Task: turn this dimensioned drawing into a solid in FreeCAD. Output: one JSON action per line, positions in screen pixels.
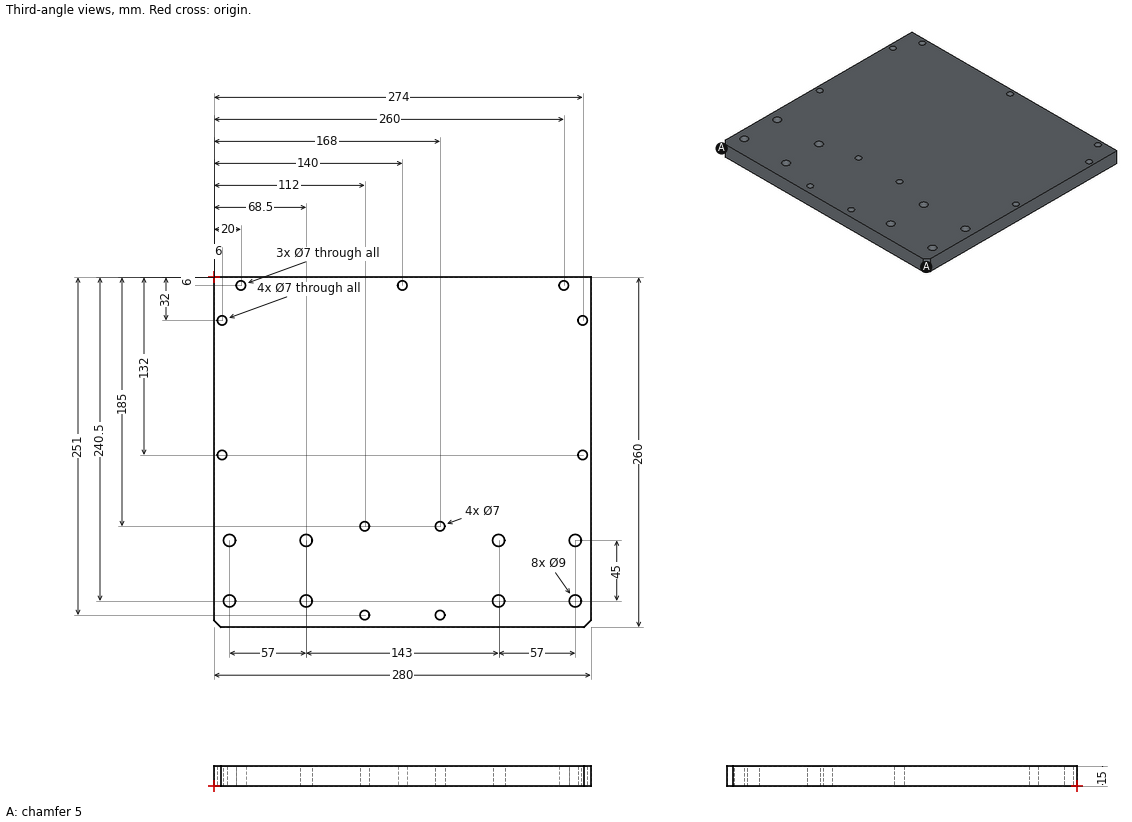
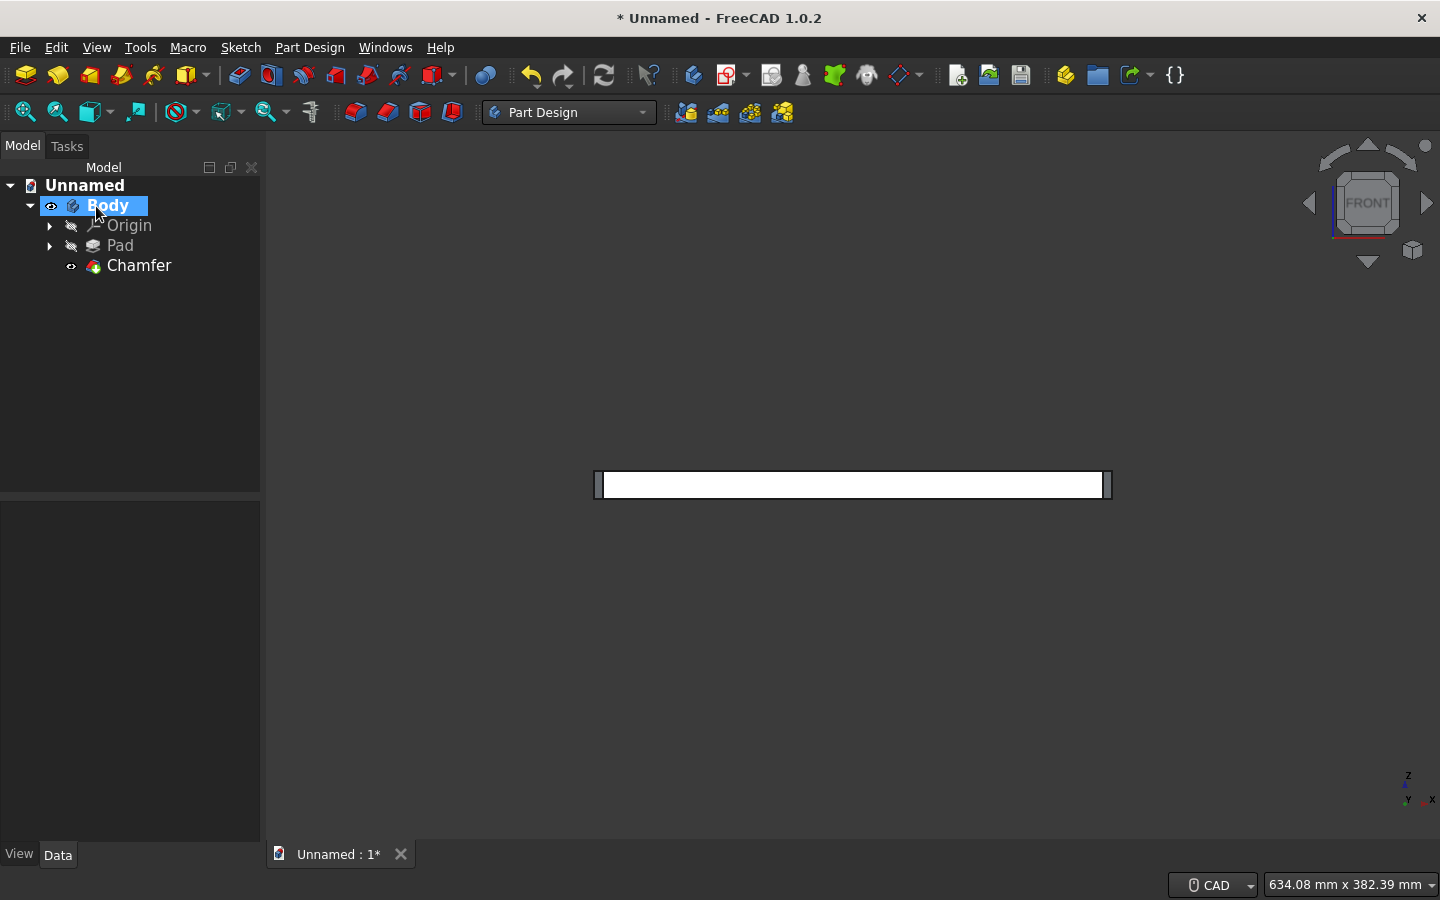
{"action": "left_click", "coordinate": [26, 112]}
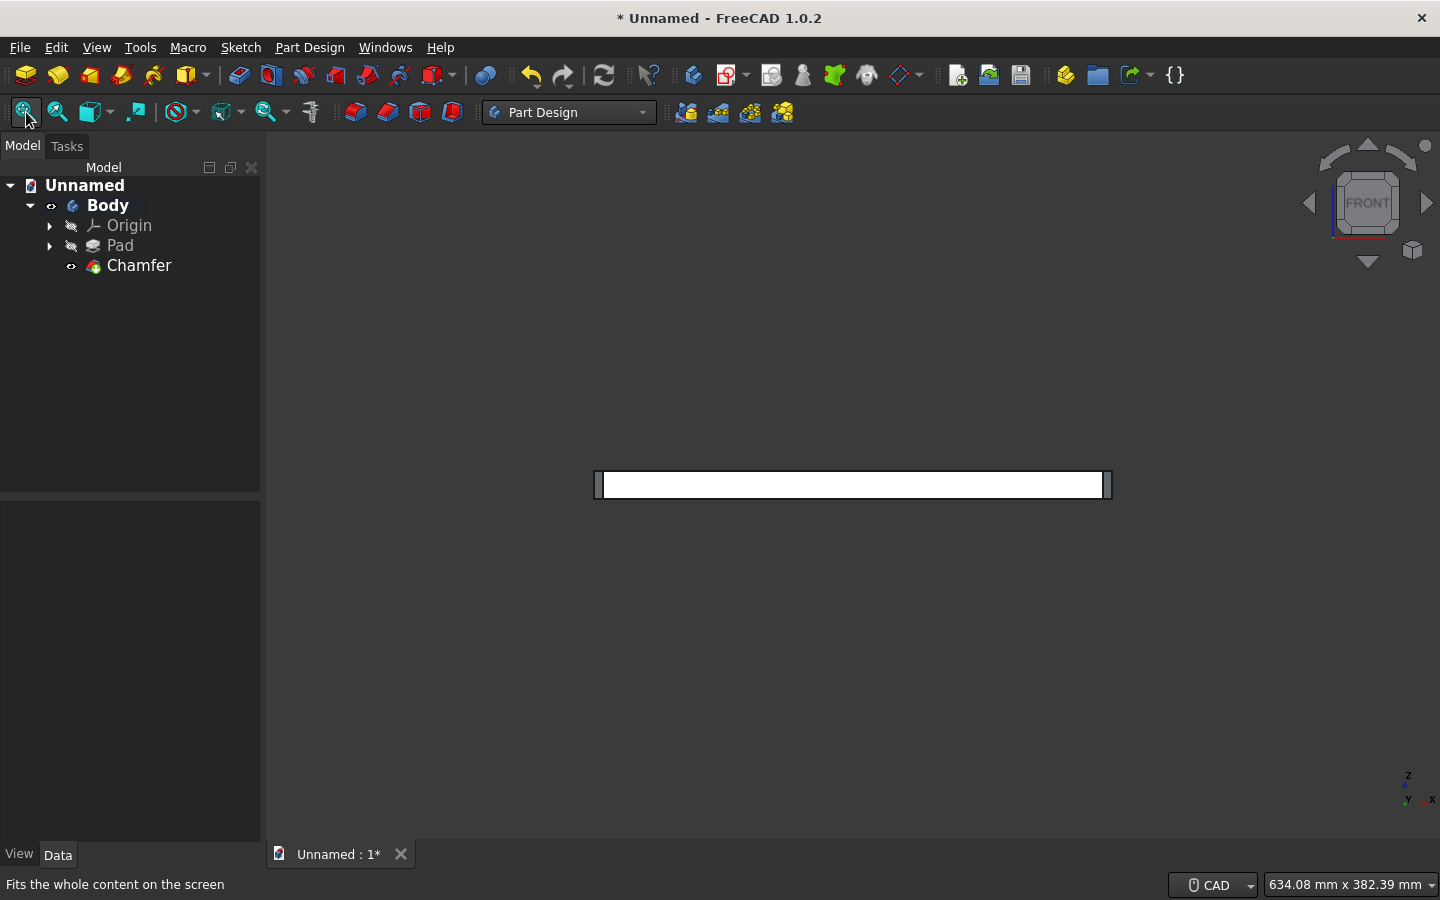
{"action": "key", "text": "5"}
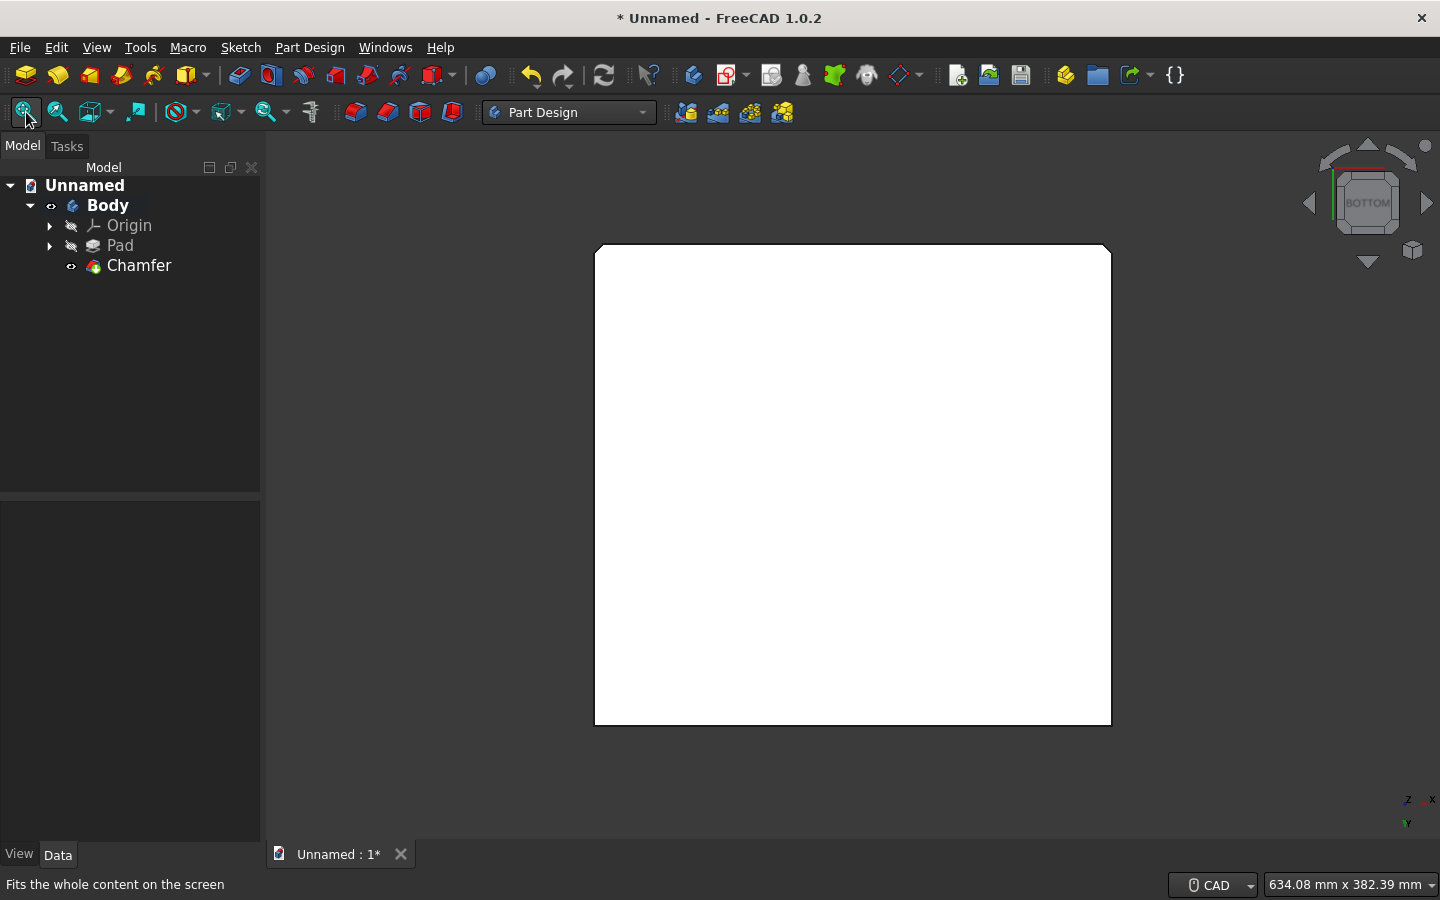
{"action": "left_click", "coordinate": [853, 484]}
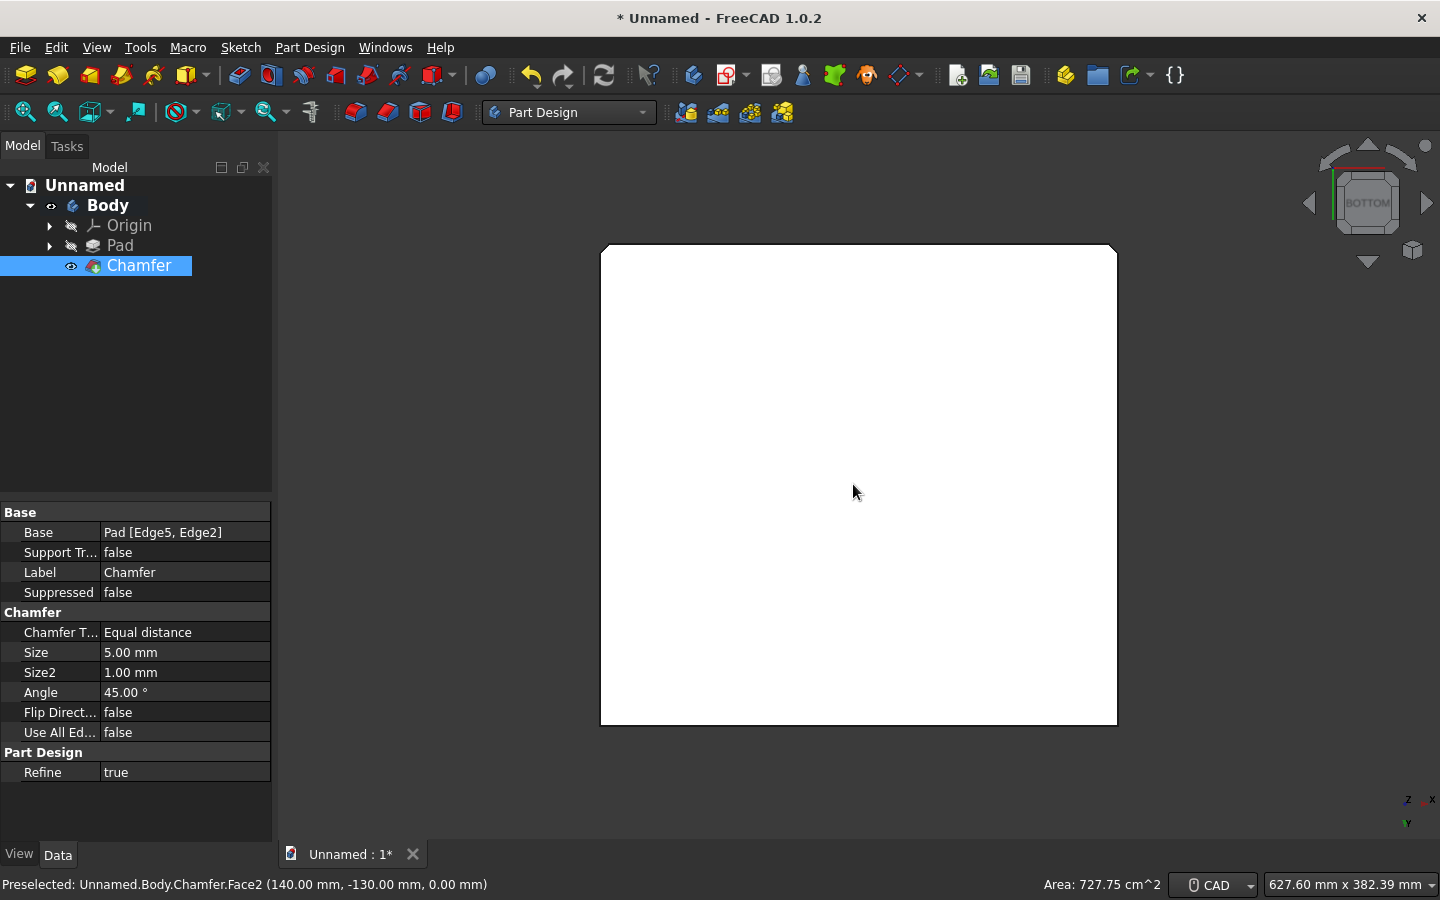
{"action": "left_click", "coordinate": [726, 76]}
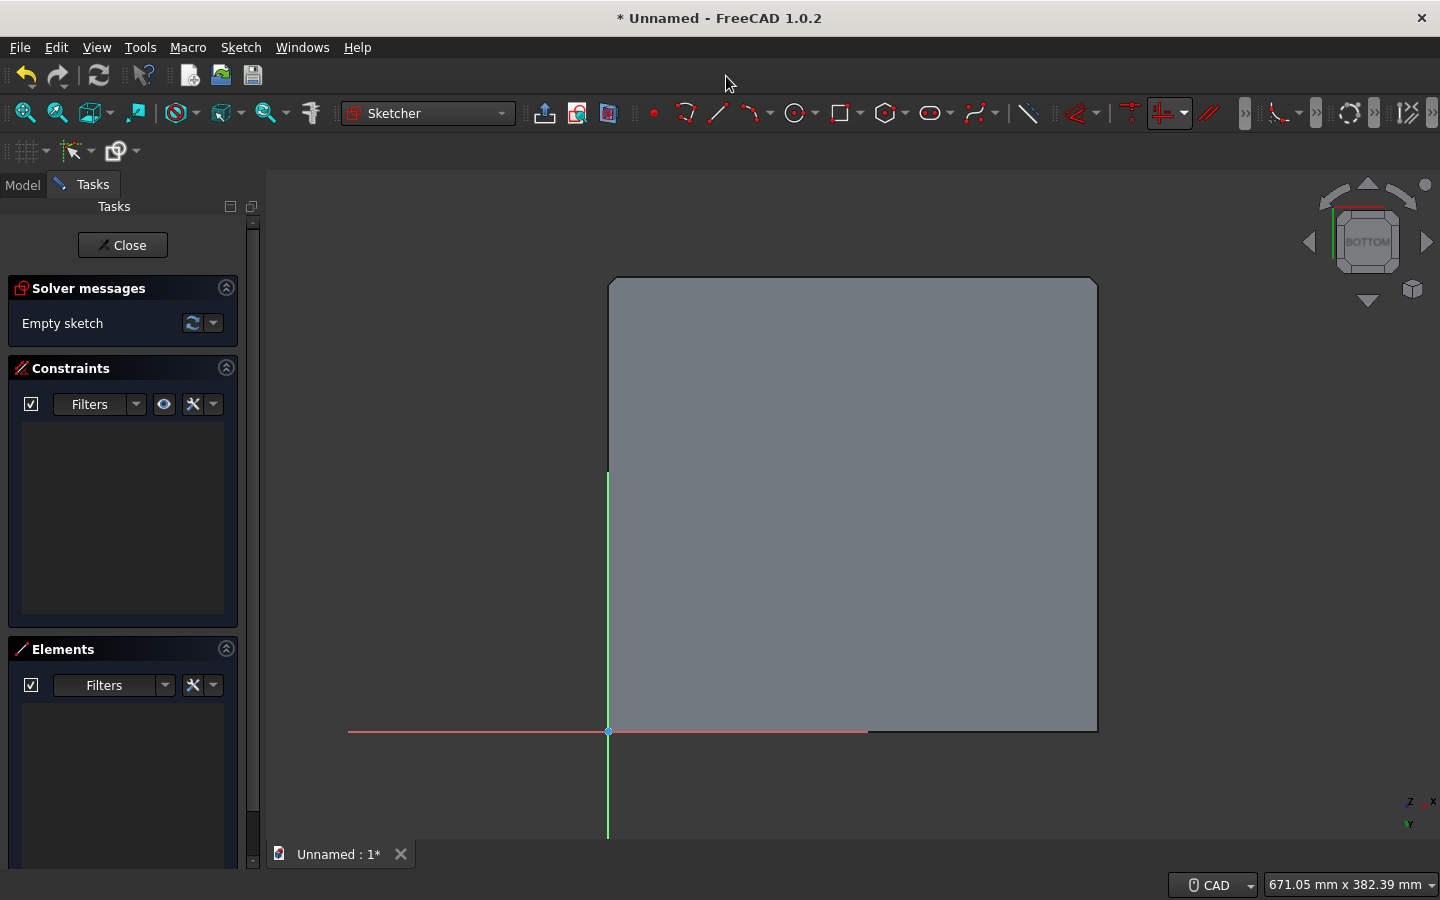
{"action": "scroll", "coordinate": [883, 284], "scroll_direction": "up", "scroll_amount": 6}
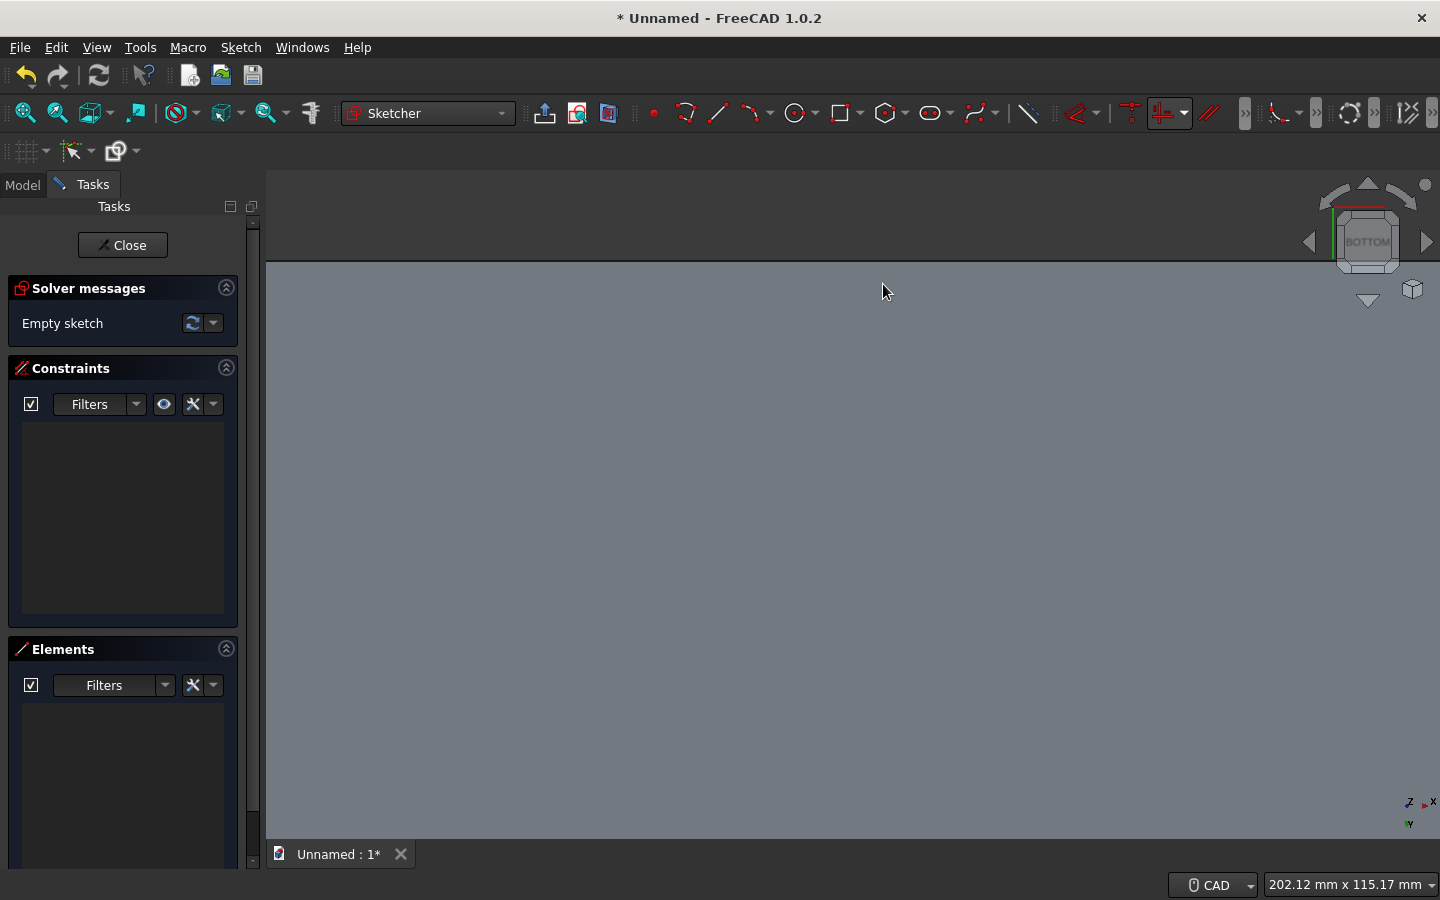
{"action": "left_click", "coordinate": [796, 114]}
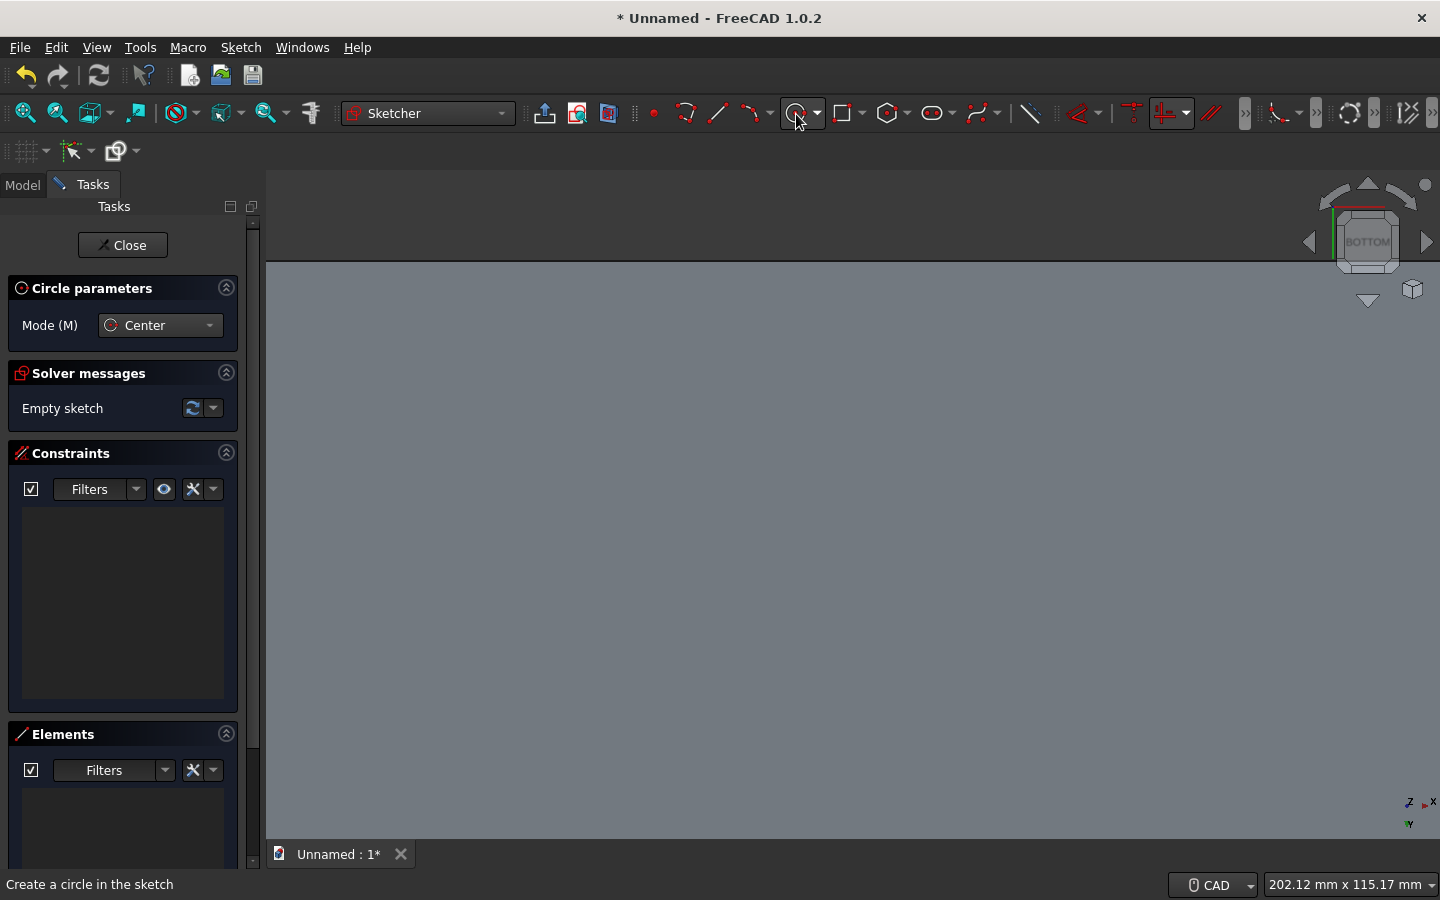
{"action": "left_click", "coordinate": [945, 696]}
{"action": "mouse_move", "coordinate": [959, 682]}